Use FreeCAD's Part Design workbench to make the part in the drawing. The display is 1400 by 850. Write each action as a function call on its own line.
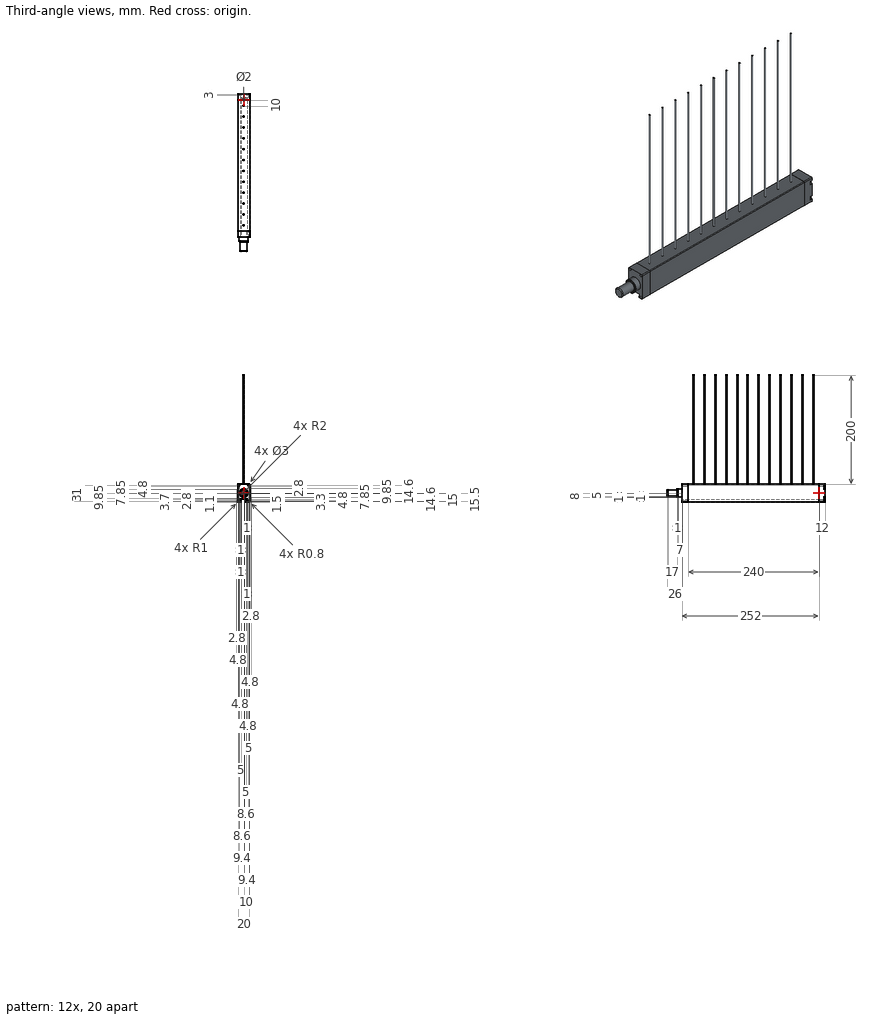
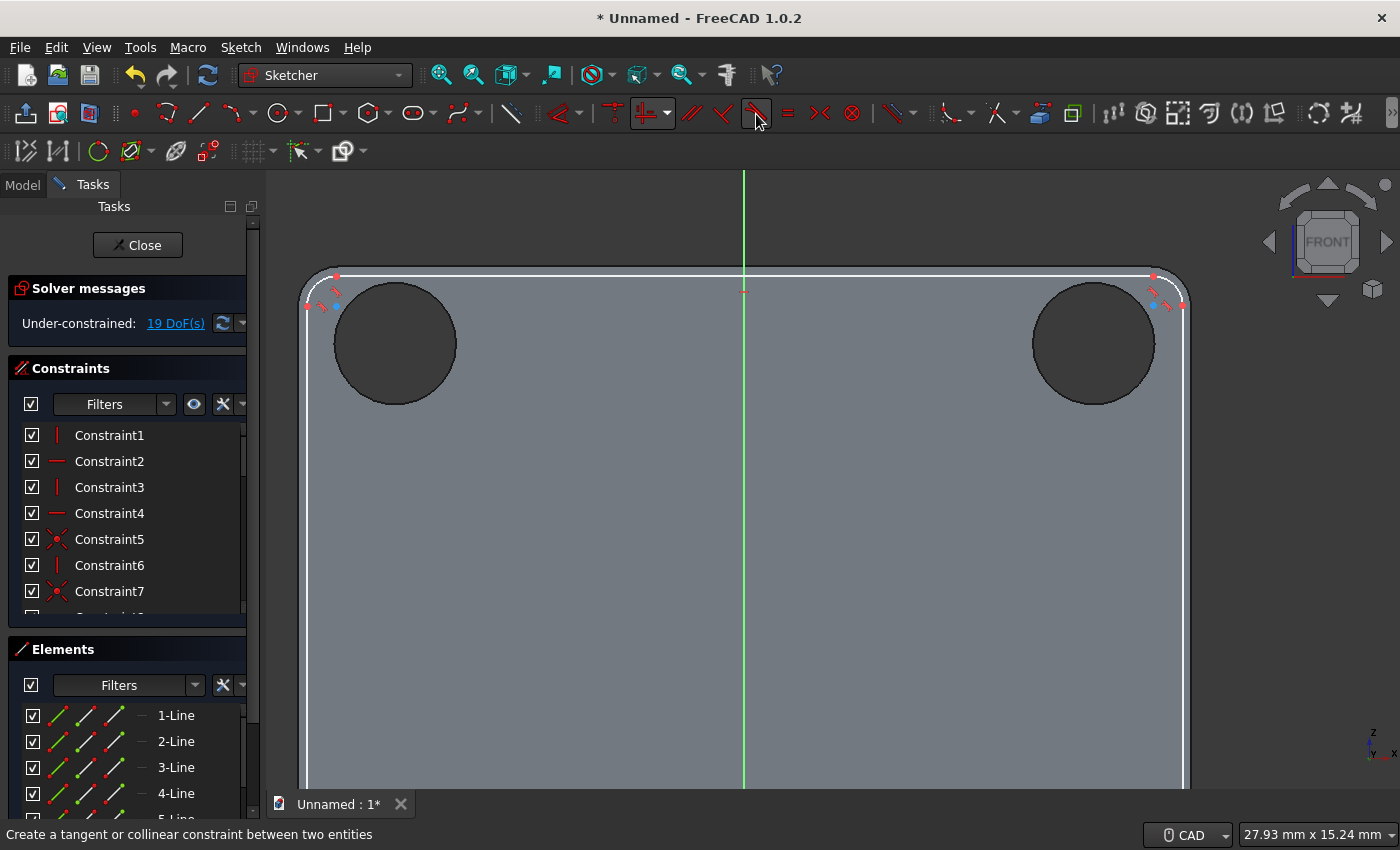
click(307, 685)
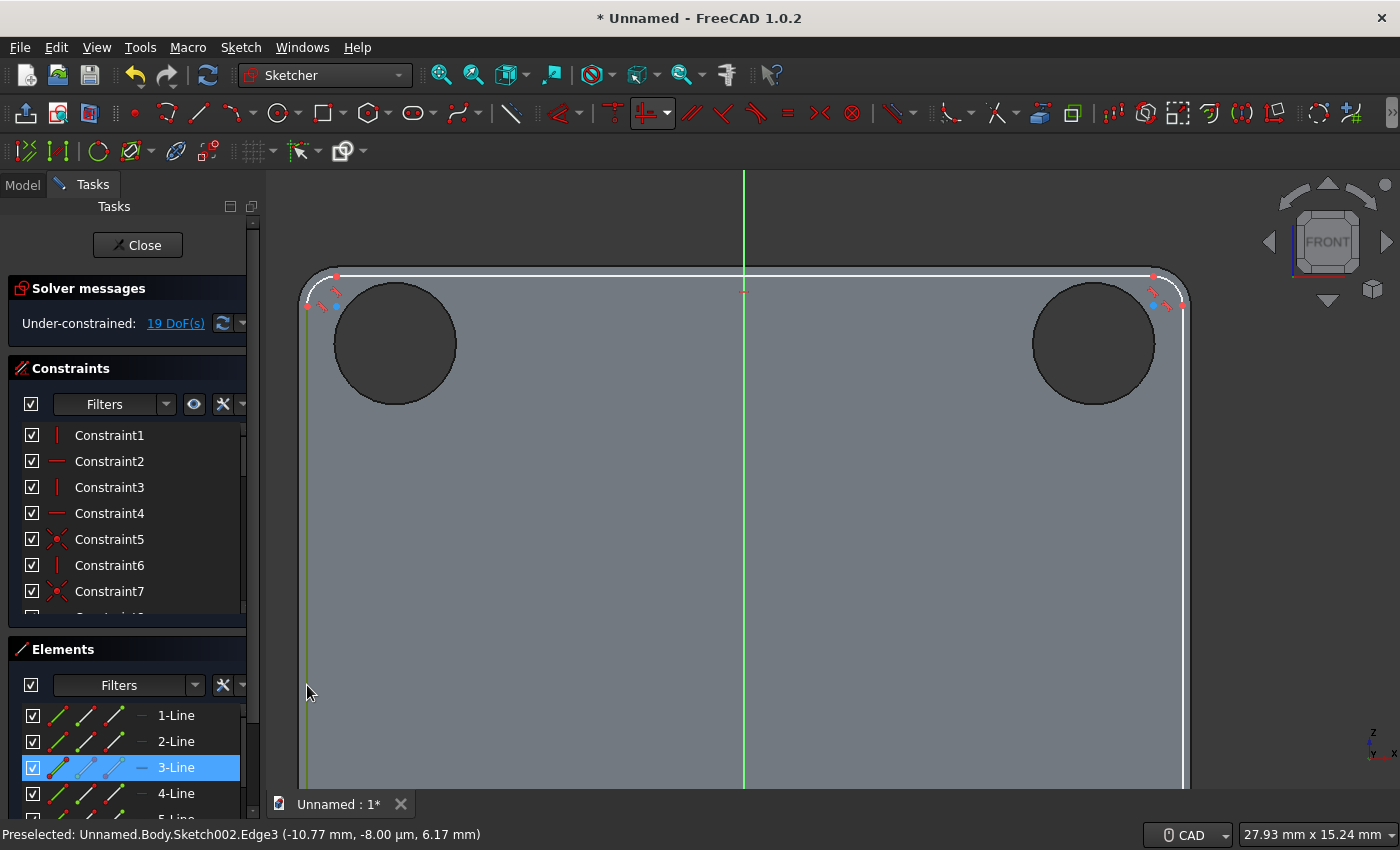
scroll(773, 283, down, 6)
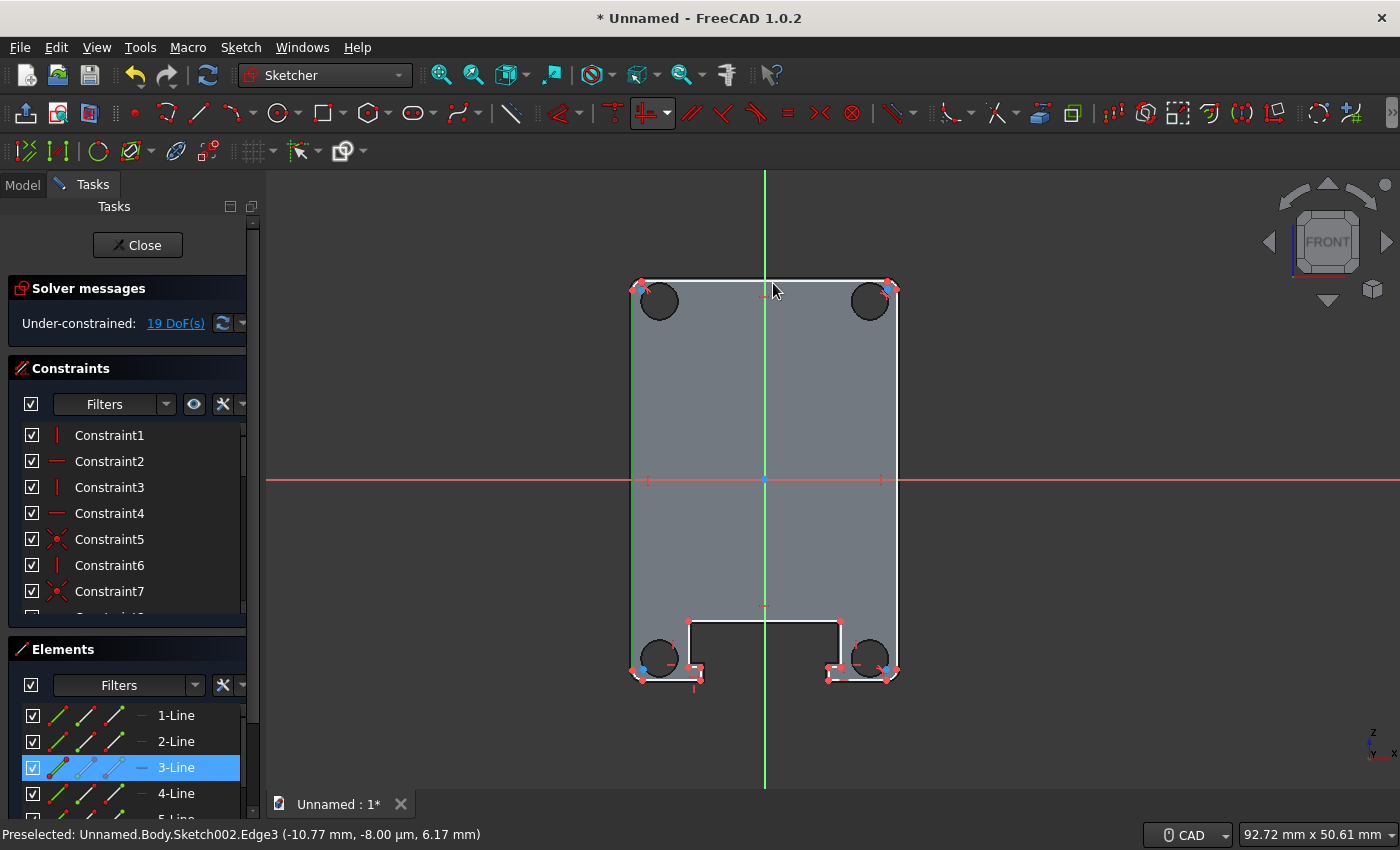
scroll(634, 675, up, 6)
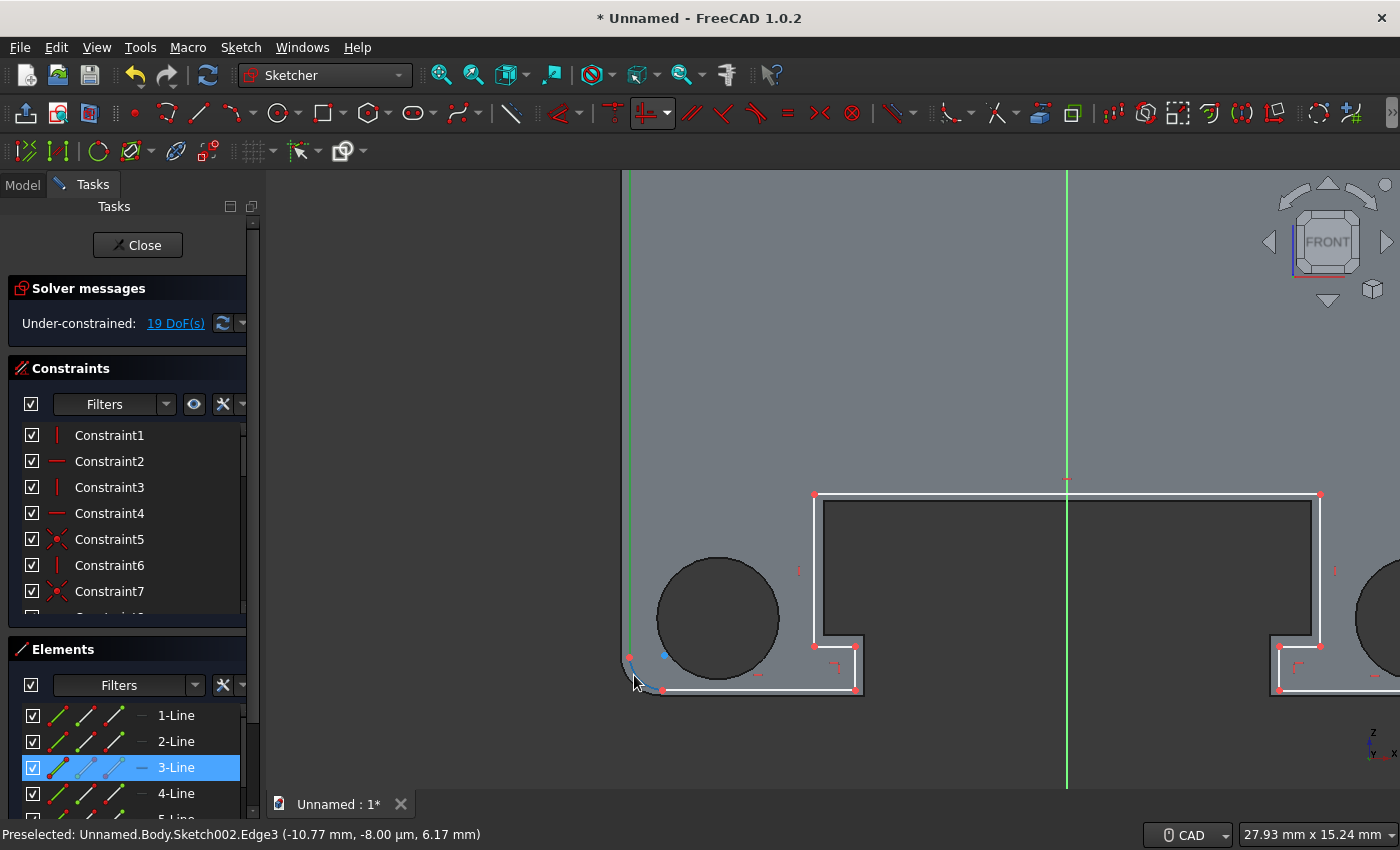
click(634, 672)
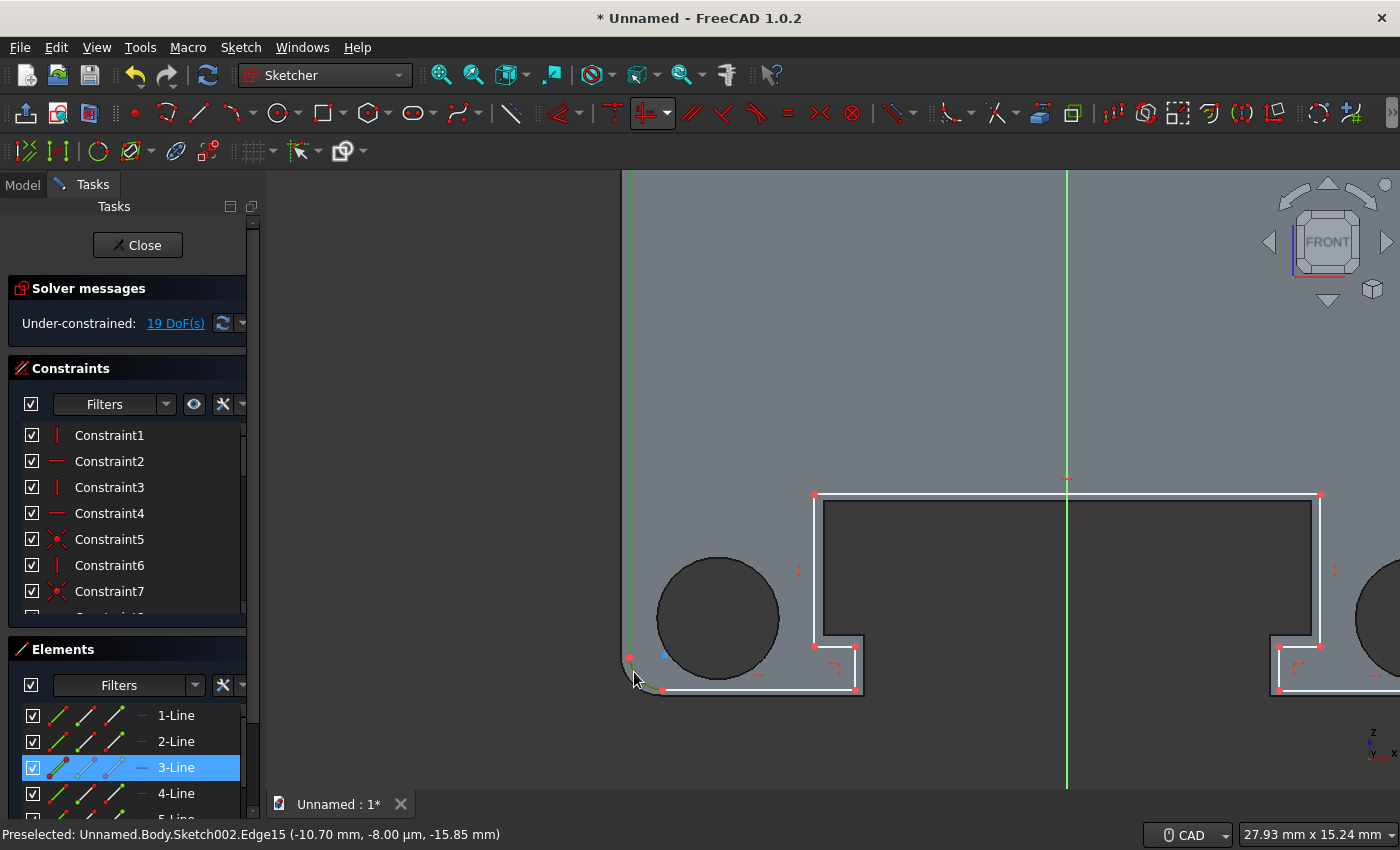
click(756, 114)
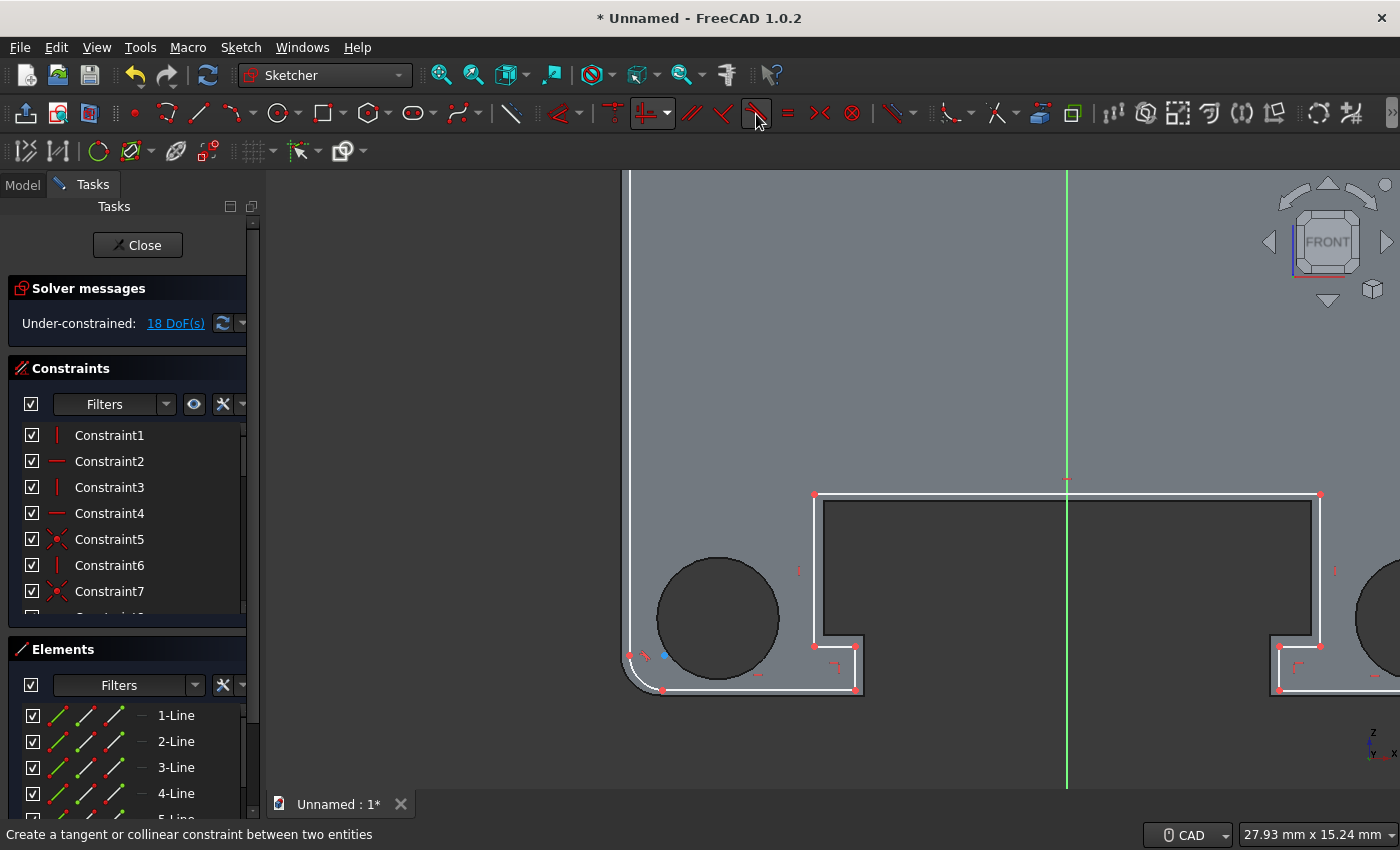
click(720, 690)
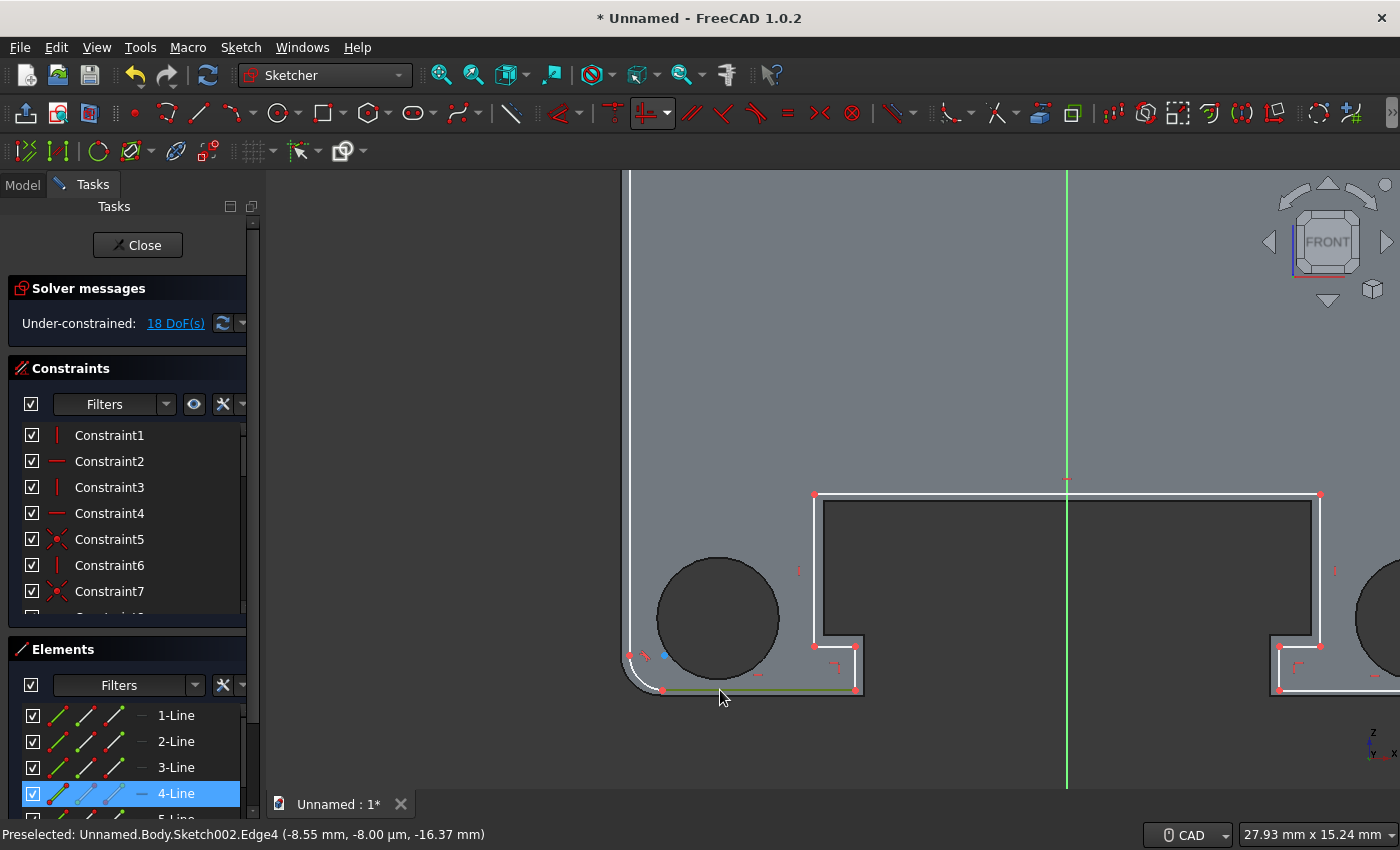
click(633, 671)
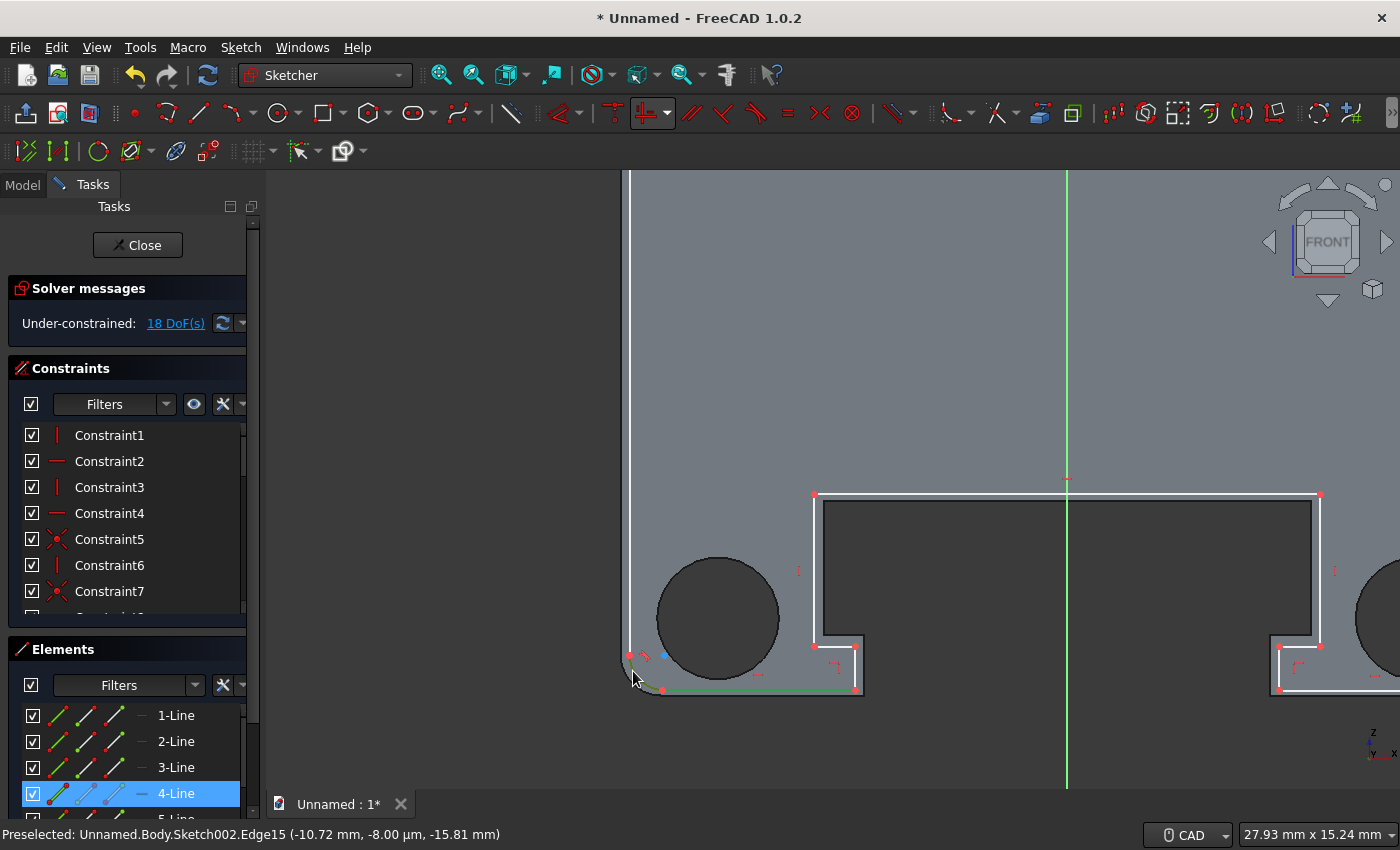
click(756, 114)